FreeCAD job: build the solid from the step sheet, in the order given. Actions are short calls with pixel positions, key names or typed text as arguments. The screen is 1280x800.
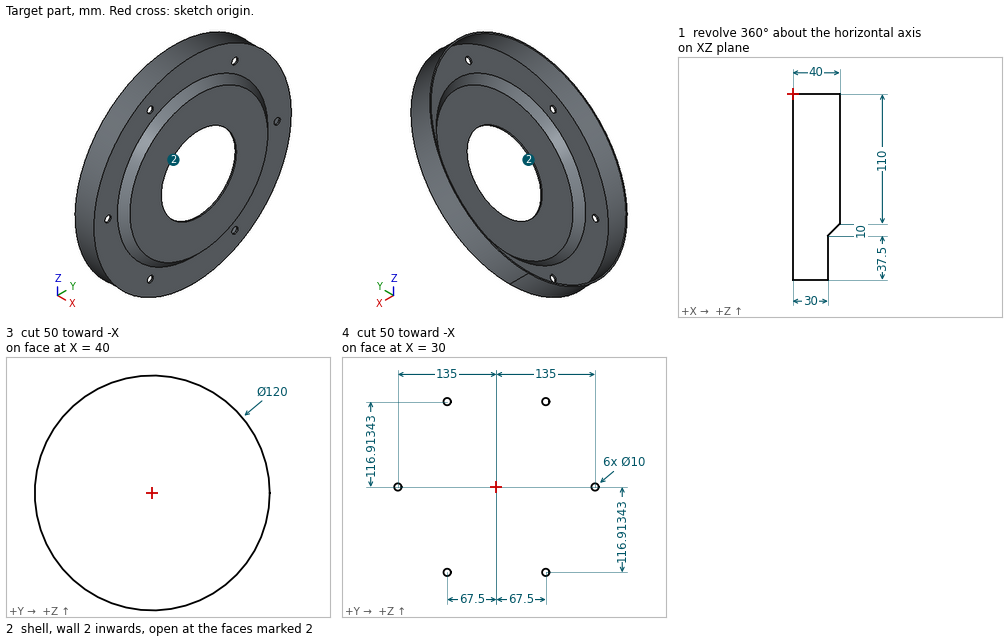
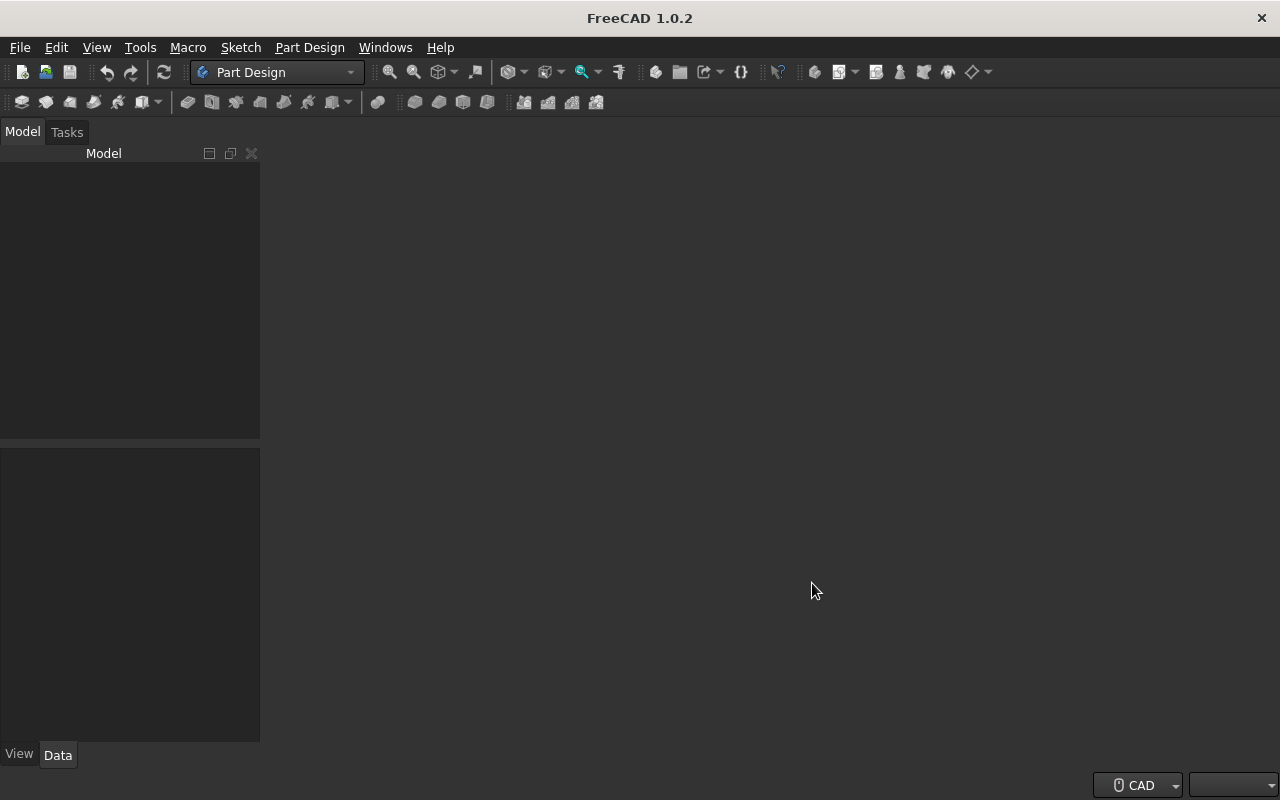
click(22, 72)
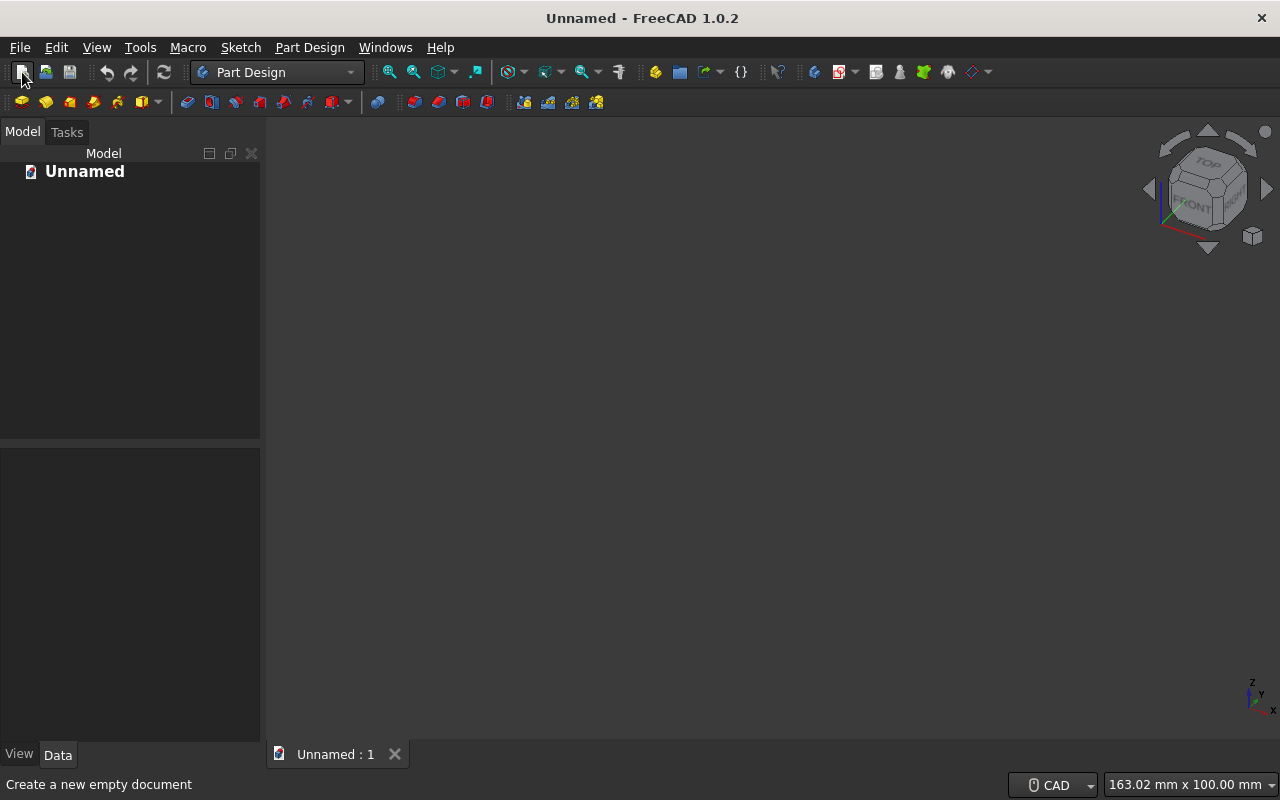
click(840, 72)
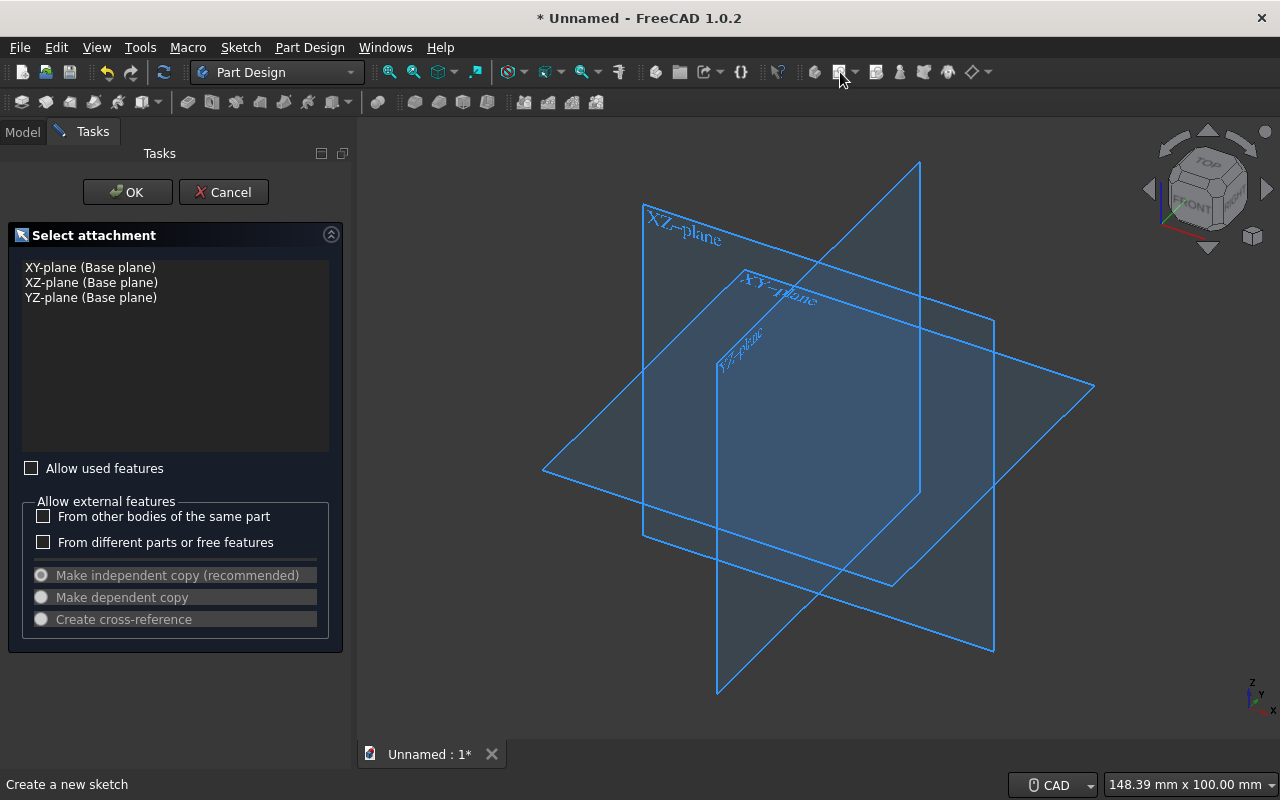
click(82, 282)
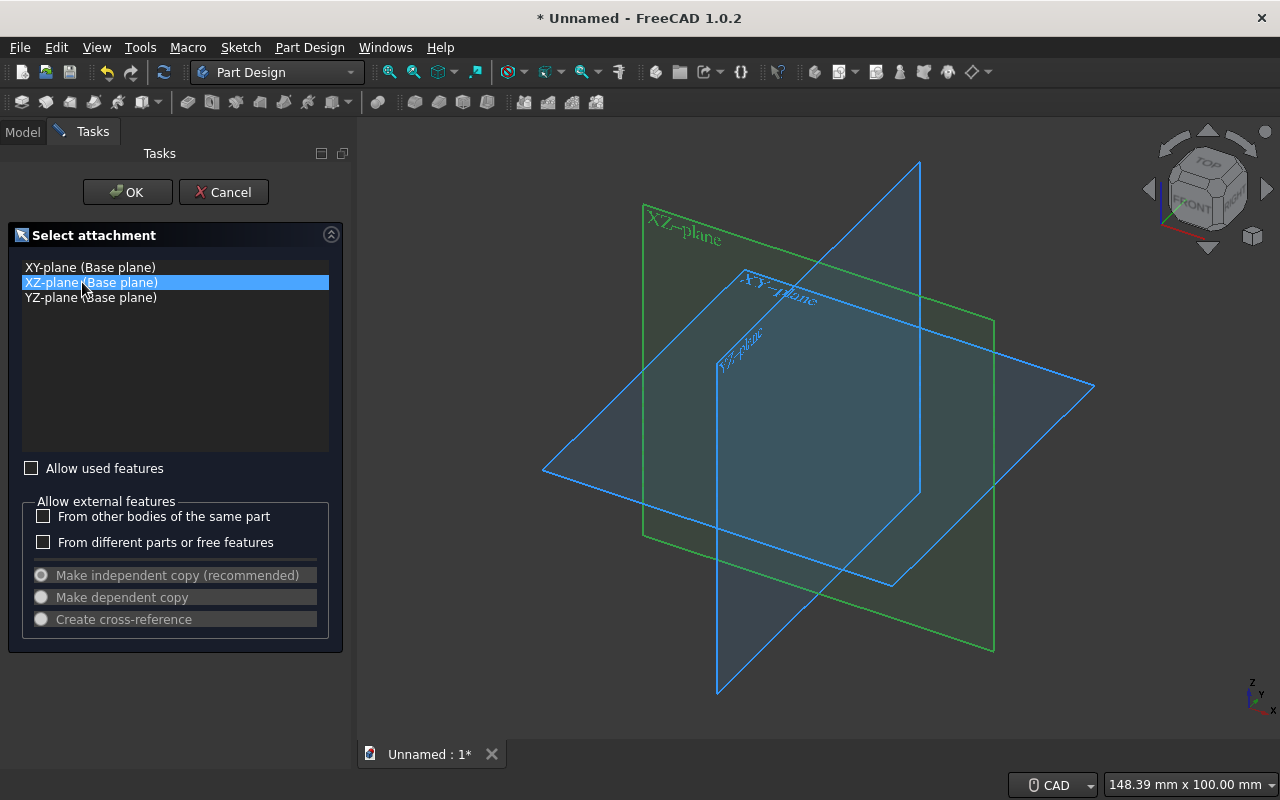
click(128, 192)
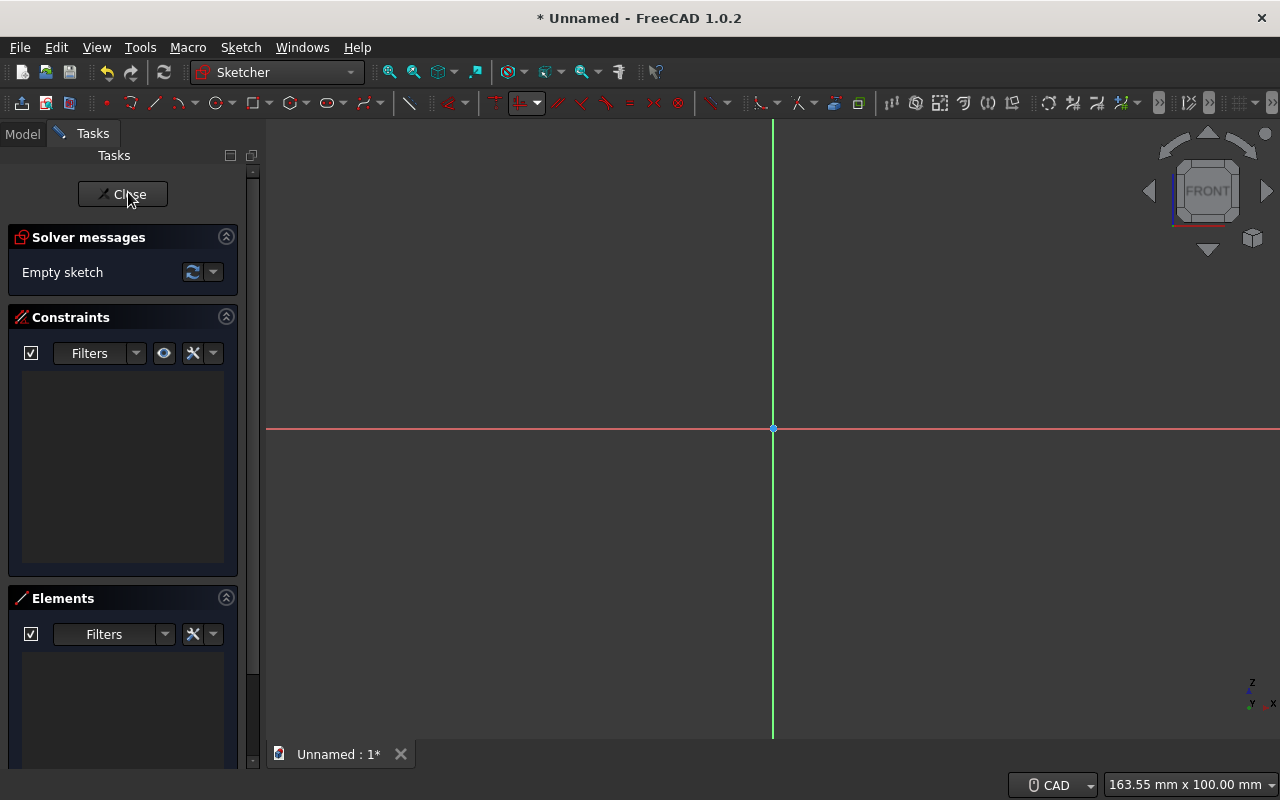
scroll(592, 147, down, 5)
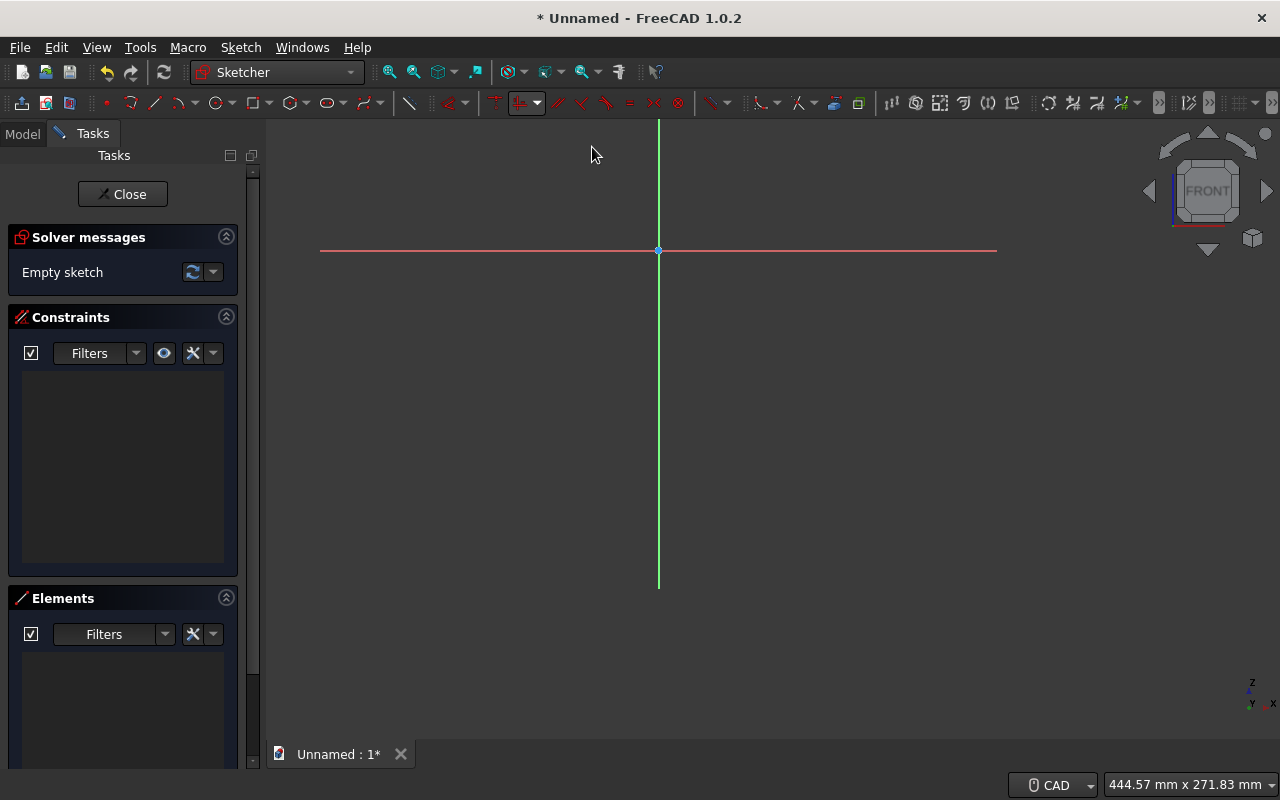
click(132, 104)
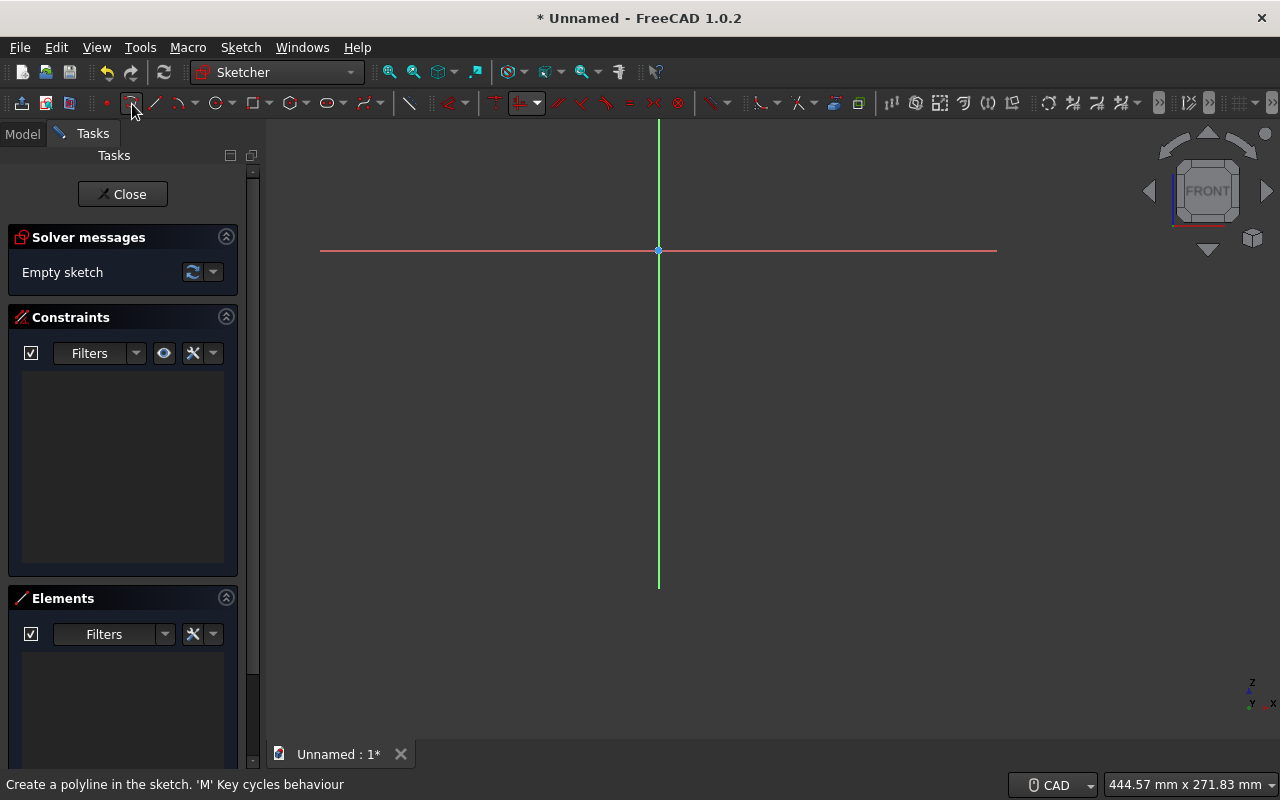
click(659, 251)
click(750, 260)
click(750, 502)
click(727, 524)
click(727, 610)
click(668, 610)
click(659, 251)
key(Escape)
key(Escape)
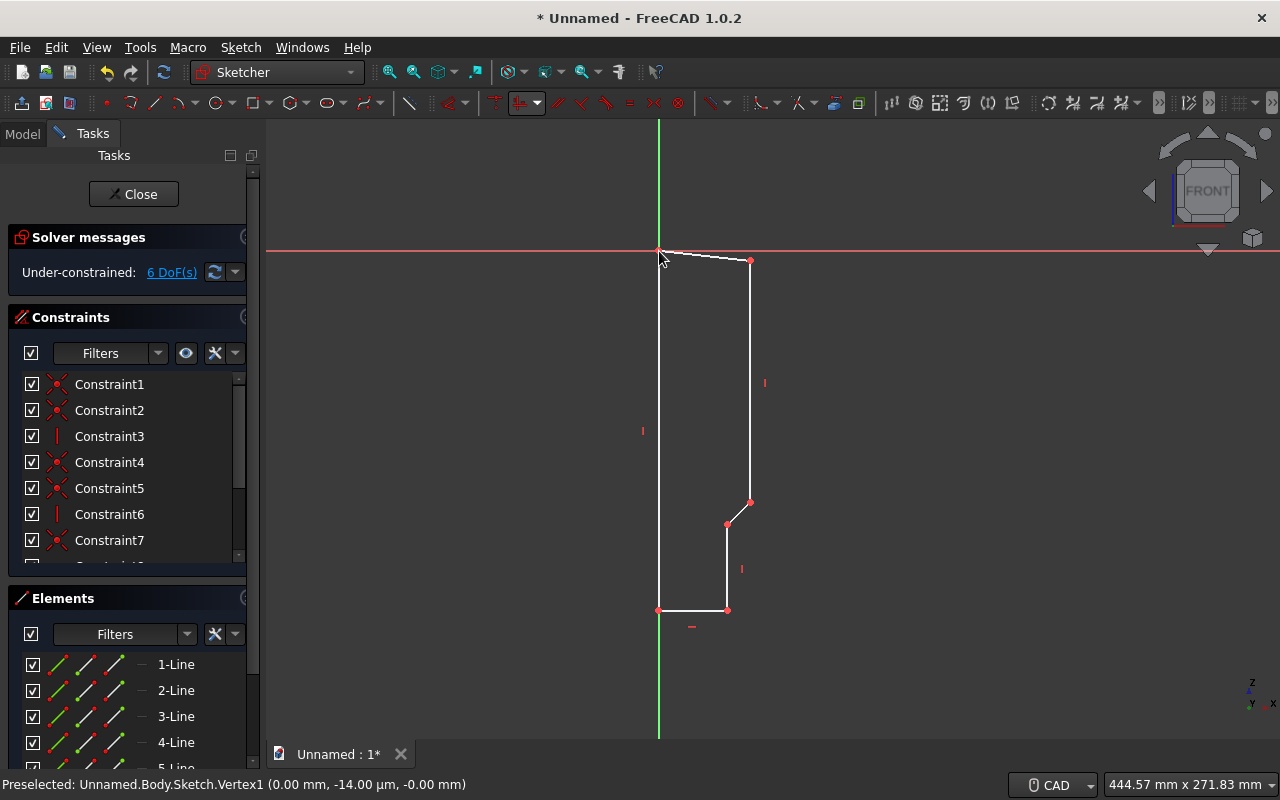
click(686, 254)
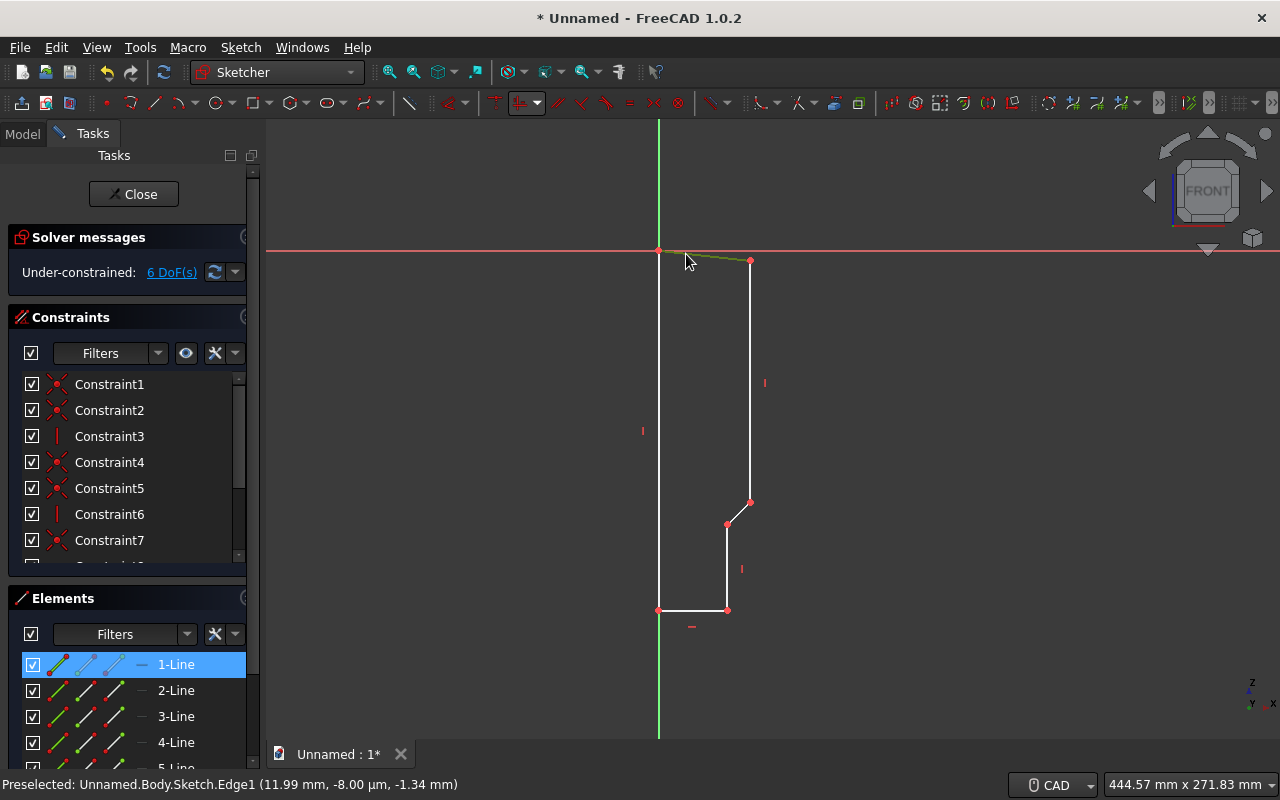
click(540, 104)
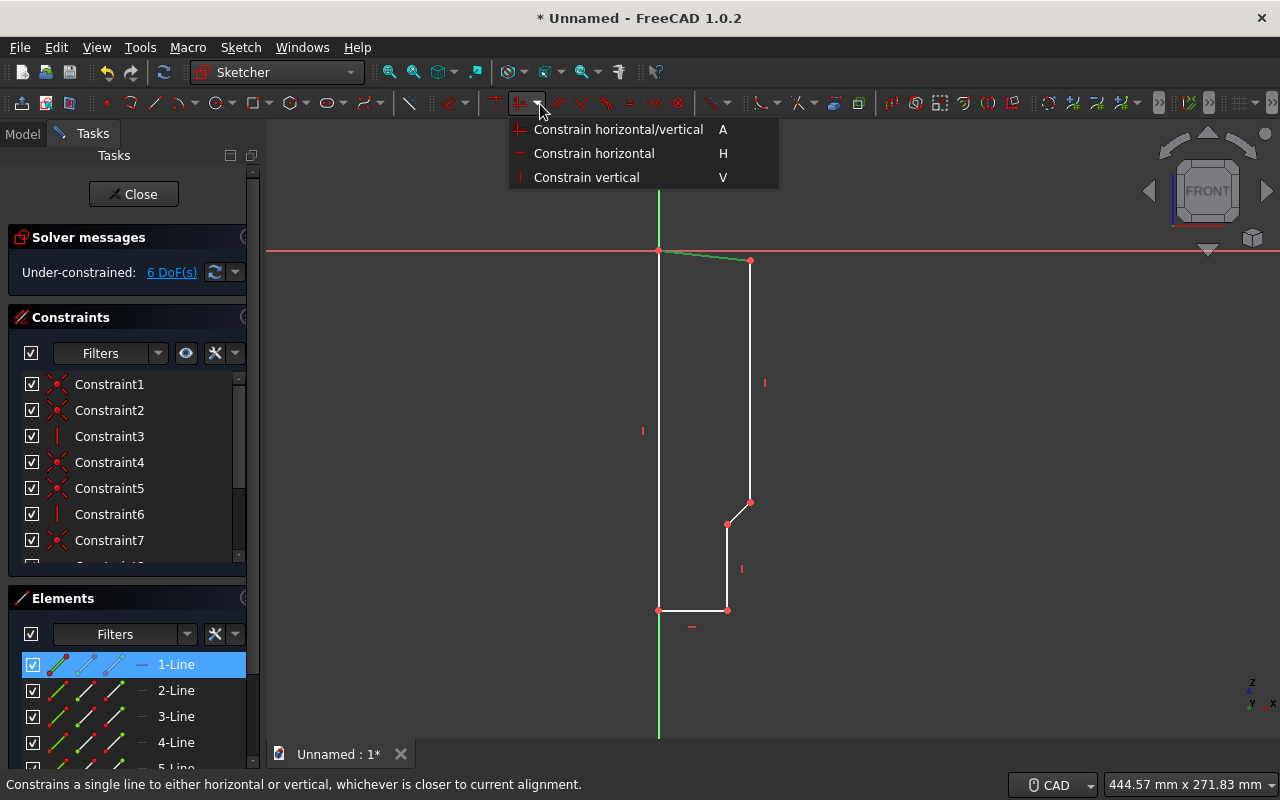
click(644, 153)